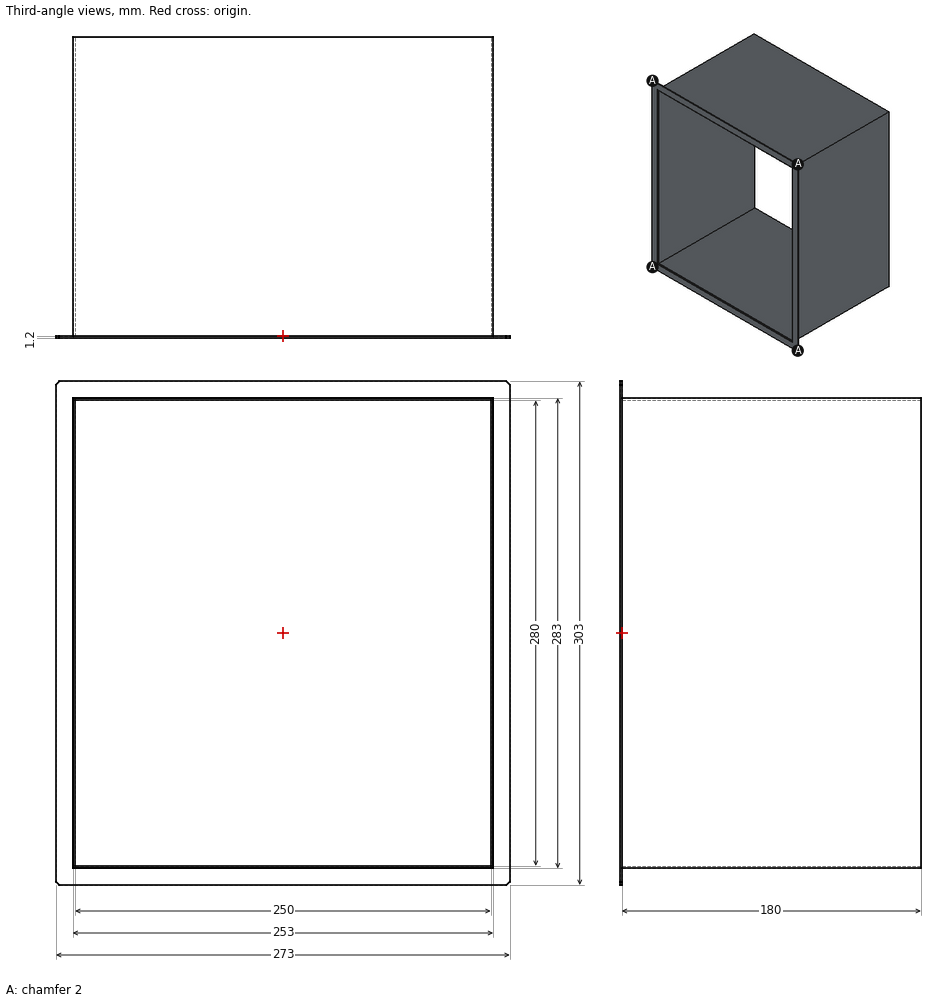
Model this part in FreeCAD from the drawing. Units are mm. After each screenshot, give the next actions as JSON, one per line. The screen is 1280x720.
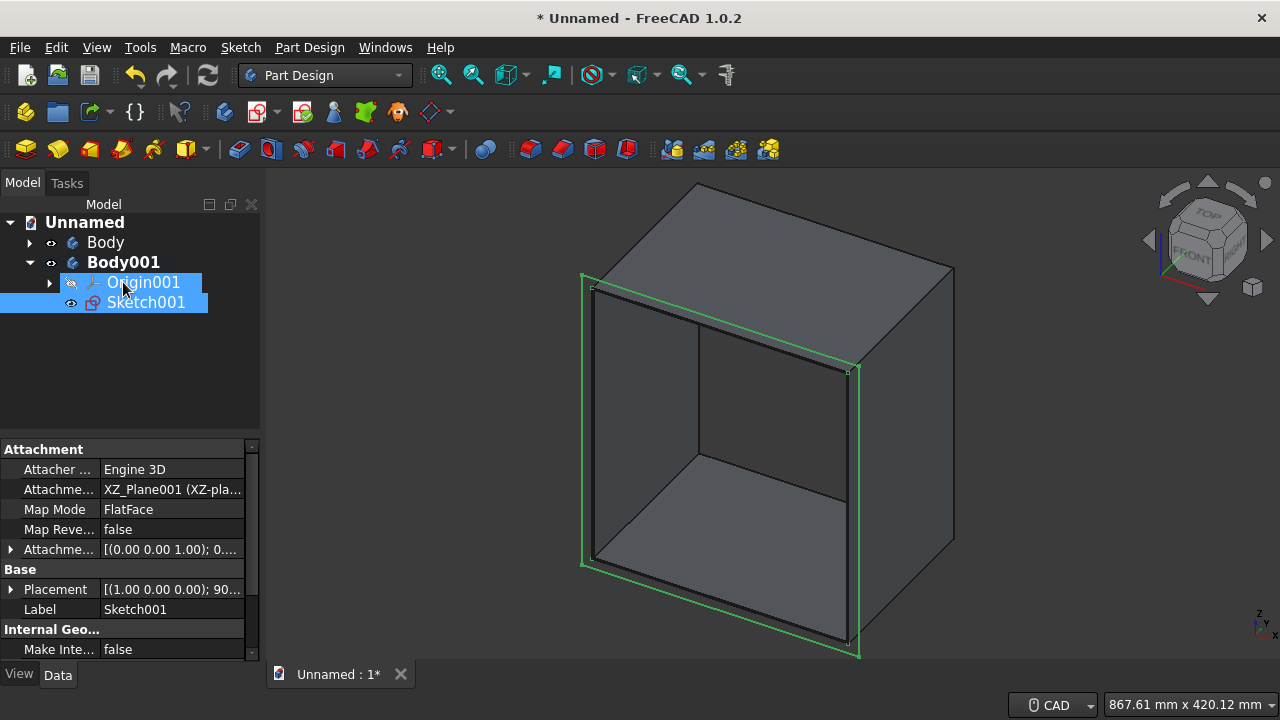
{"action": "left_click", "coordinate": [26, 150]}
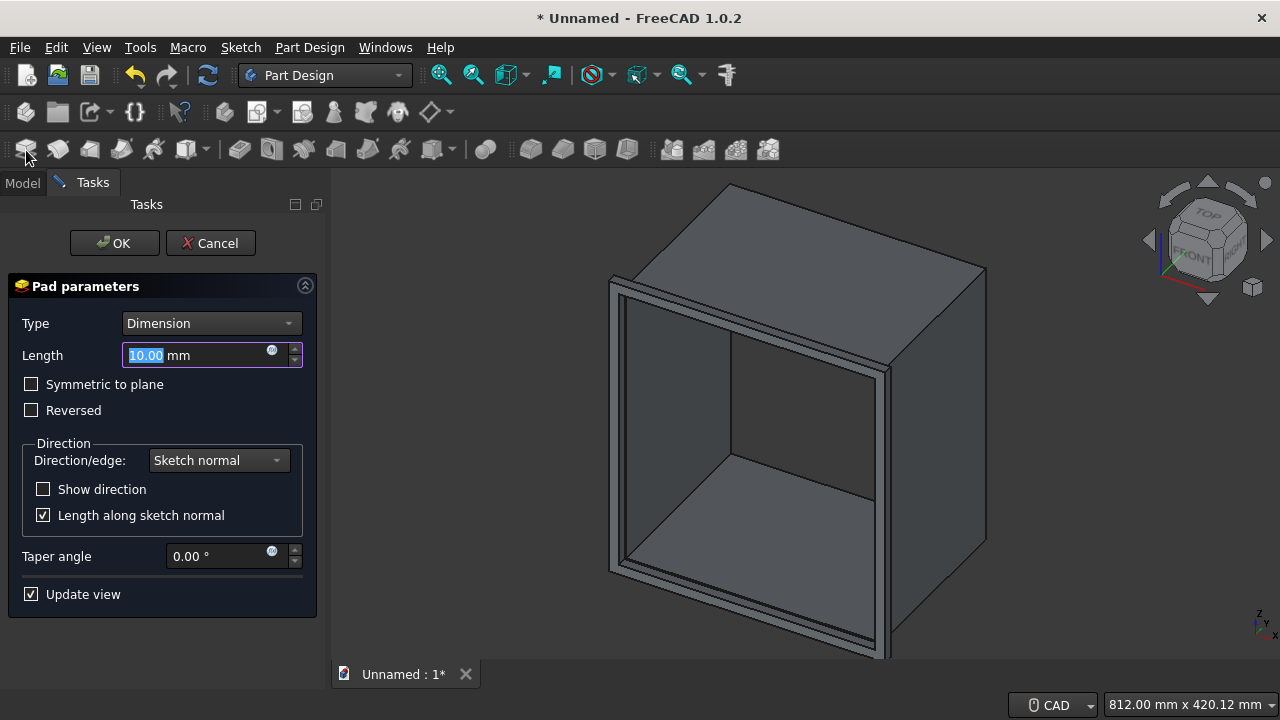
{"action": "type", "text": "1.2"}
{"action": "key", "text": "Tab"}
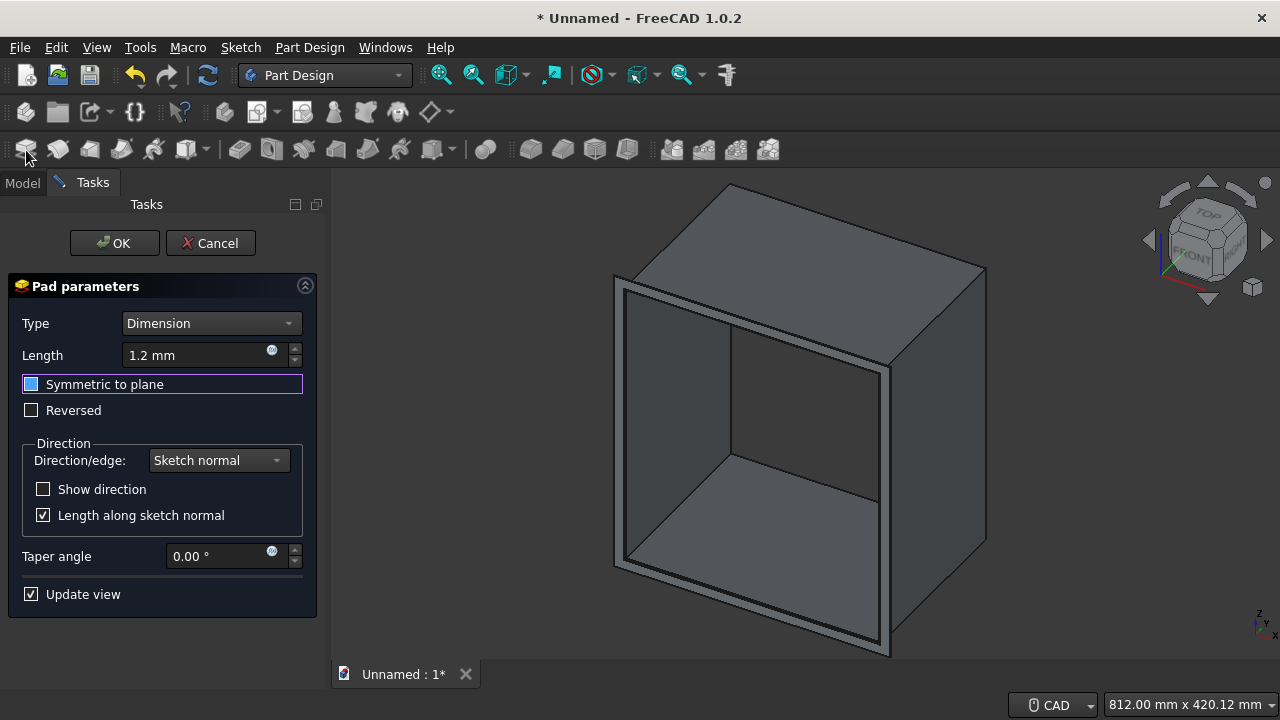
{"action": "left_click", "coordinate": [115, 243]}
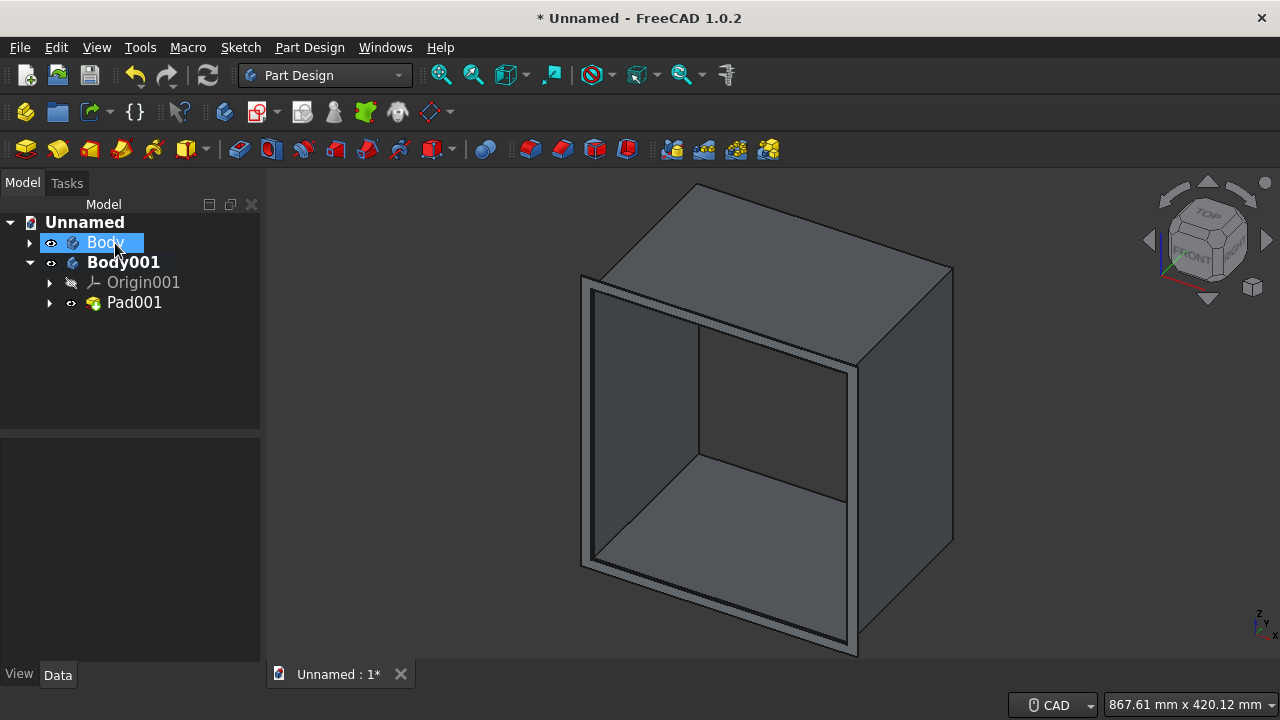
{"action": "scroll", "coordinate": [582, 565], "scroll_direction": "up", "scroll_amount": 15}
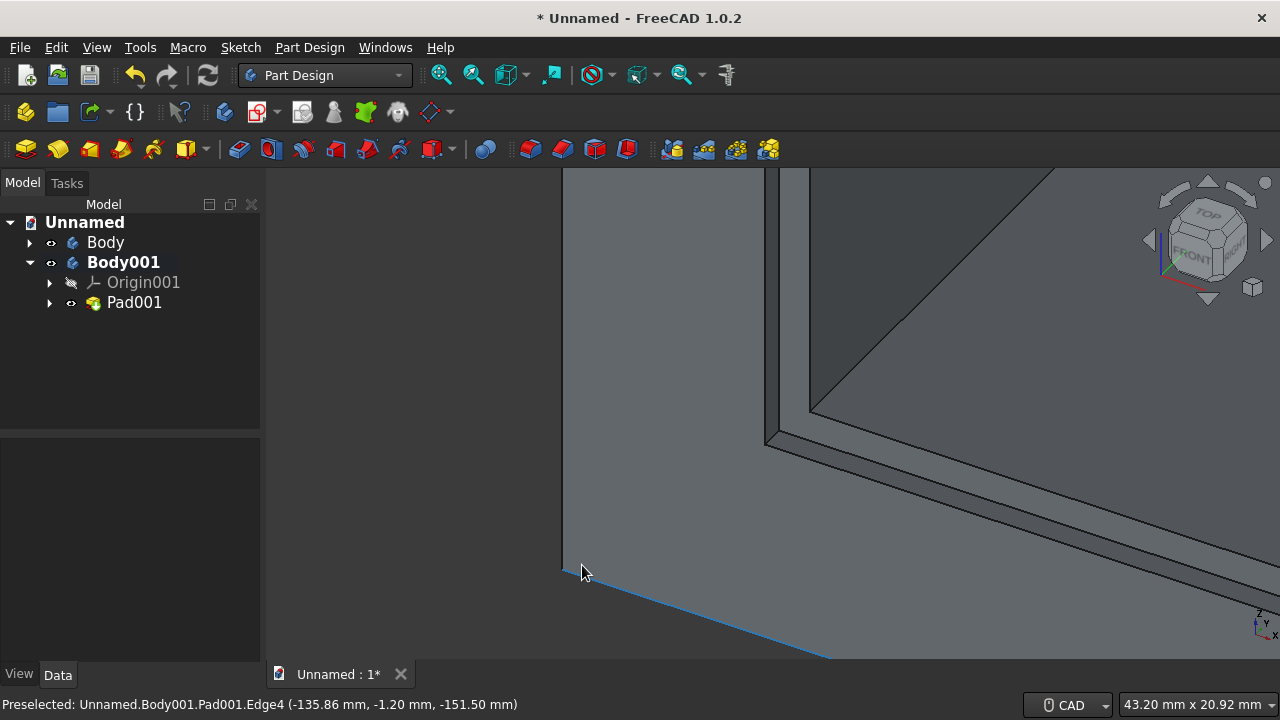
{"action": "left_click", "coordinate": [442, 76]}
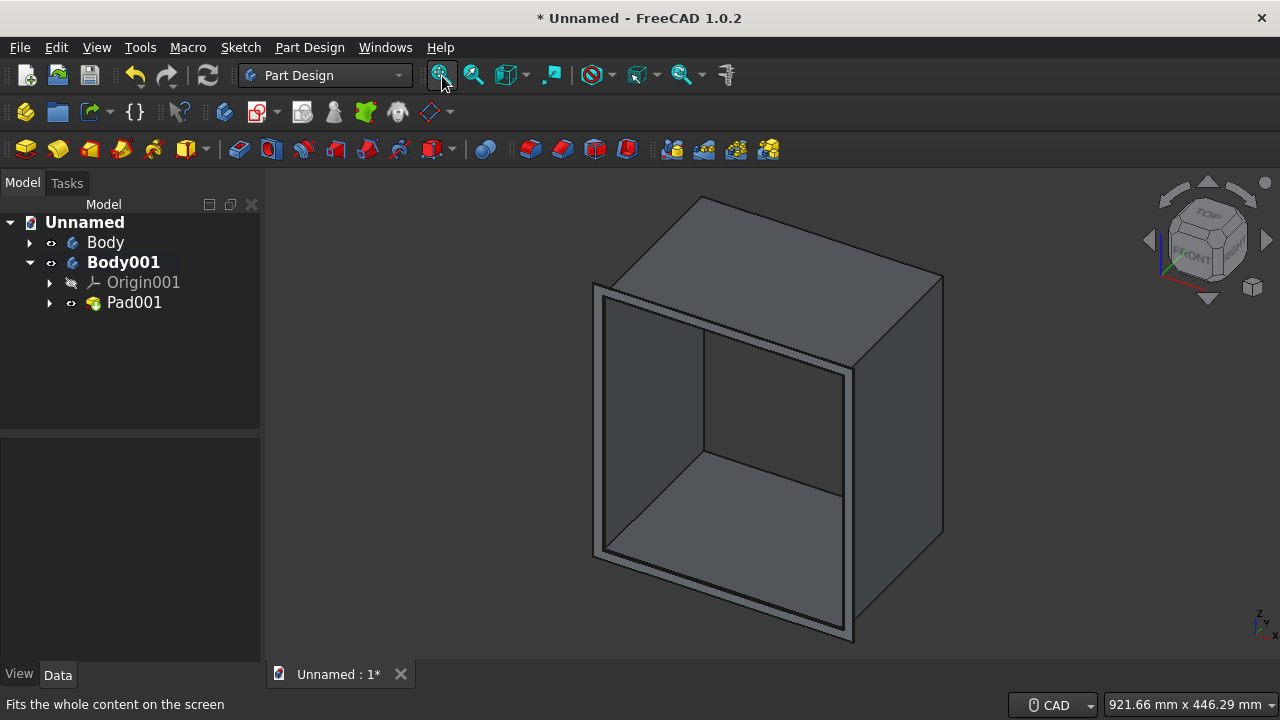
{"action": "key", "text": "0"}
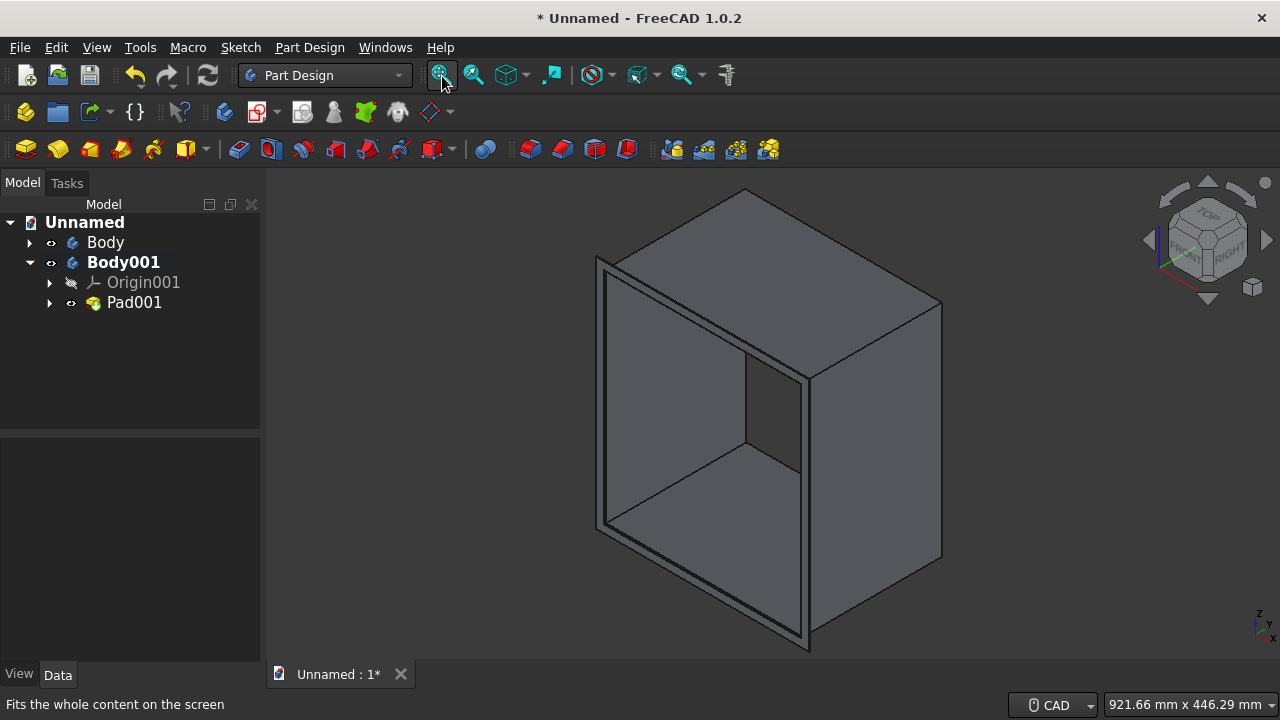
{"action": "scroll", "coordinate": [597, 528], "scroll_direction": "up", "scroll_amount": 15}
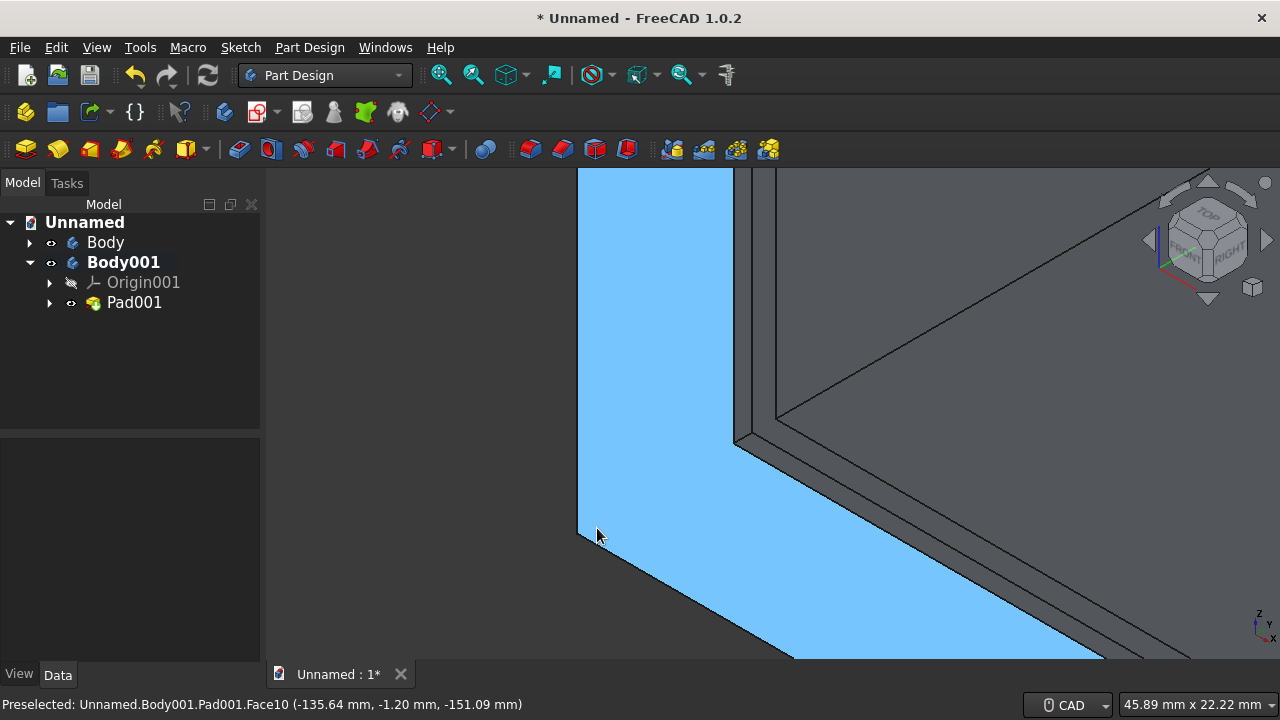
{"action": "key", "text": "v f"}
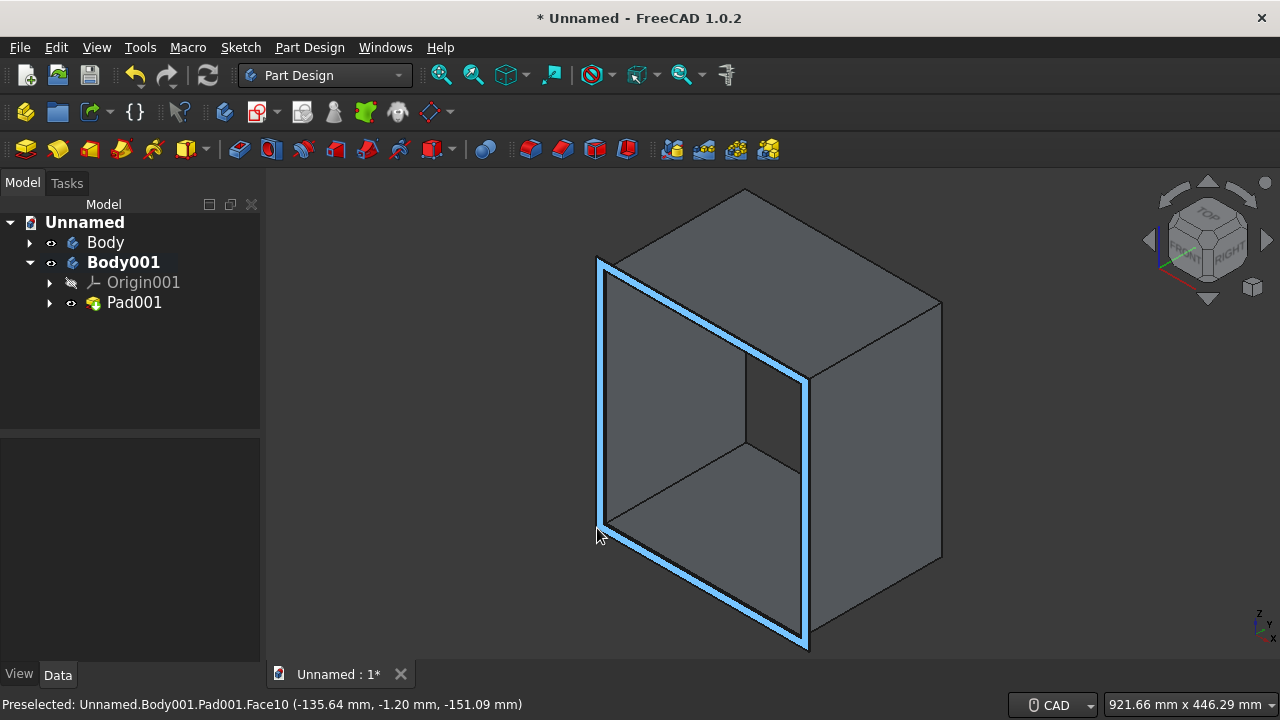
{"action": "key", "text": "2"}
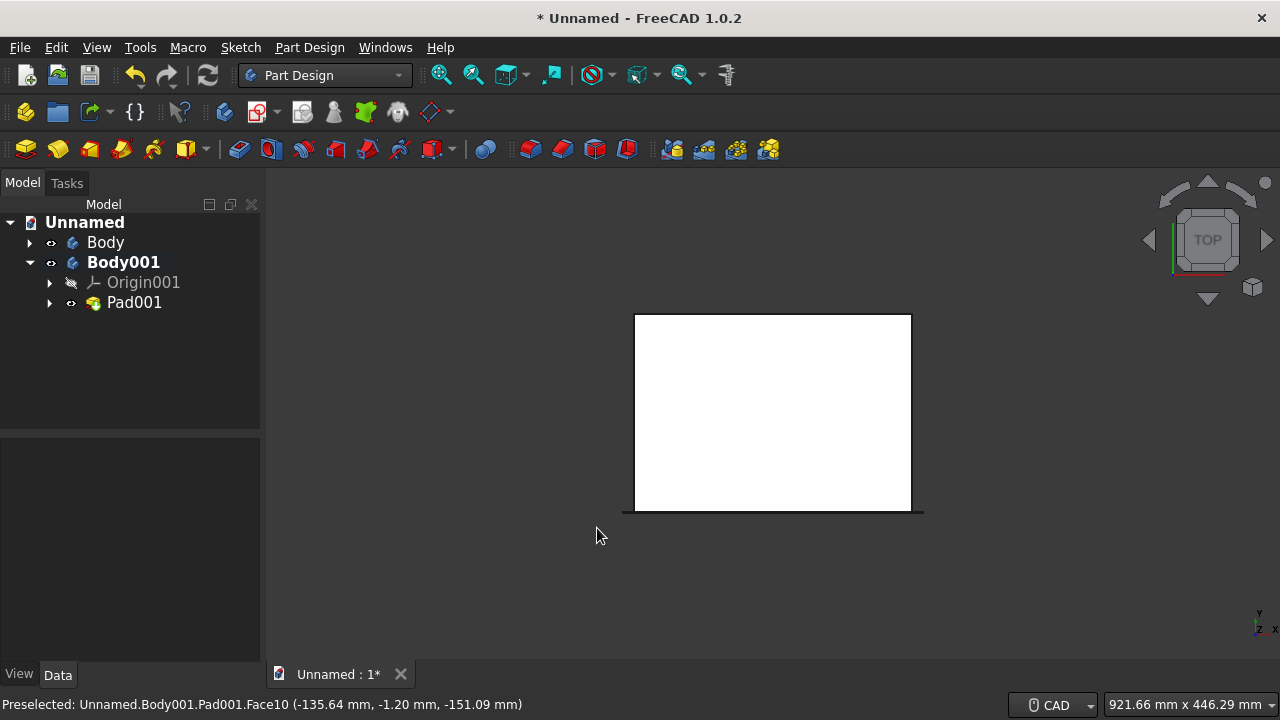
{"action": "key", "text": "v f"}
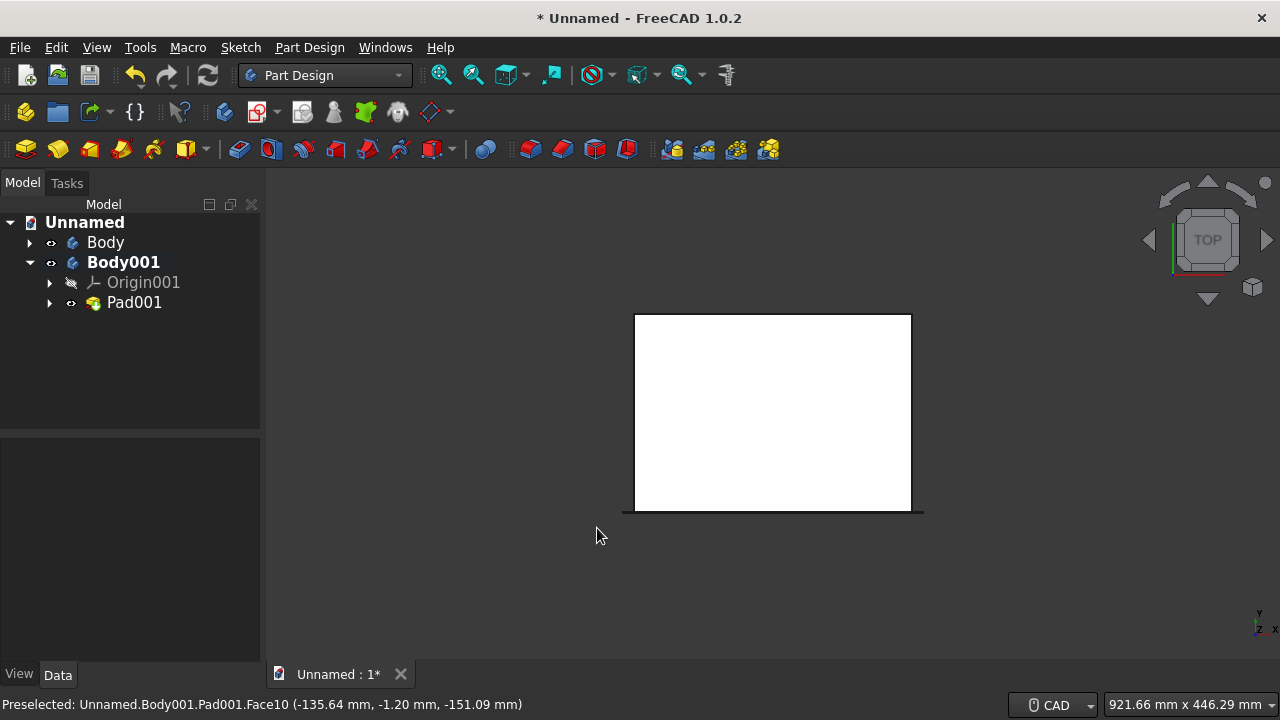
{"action": "scroll", "coordinate": [623, 512], "scroll_direction": "up", "scroll_amount": 15}